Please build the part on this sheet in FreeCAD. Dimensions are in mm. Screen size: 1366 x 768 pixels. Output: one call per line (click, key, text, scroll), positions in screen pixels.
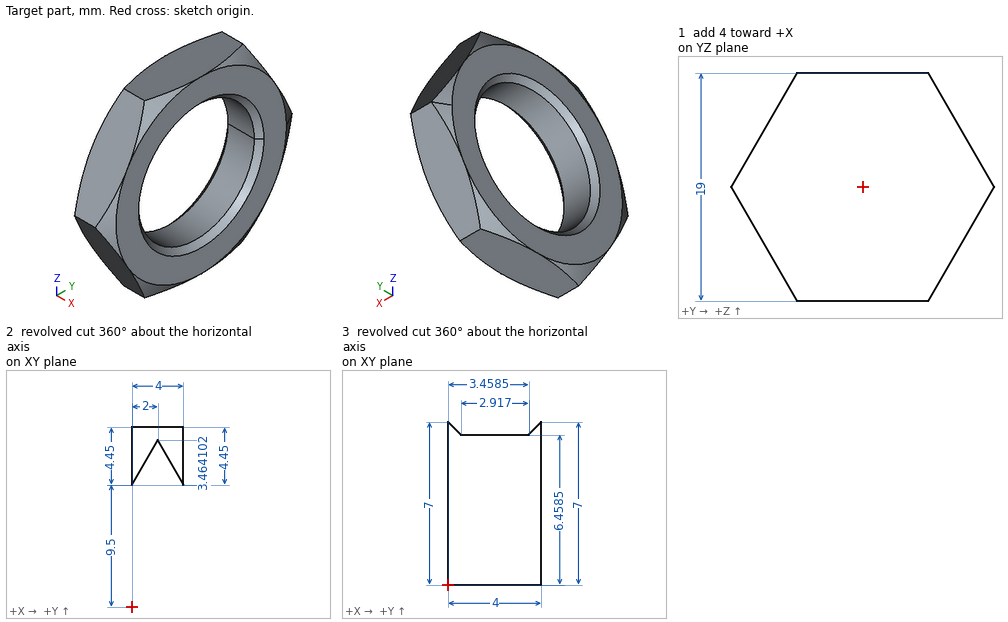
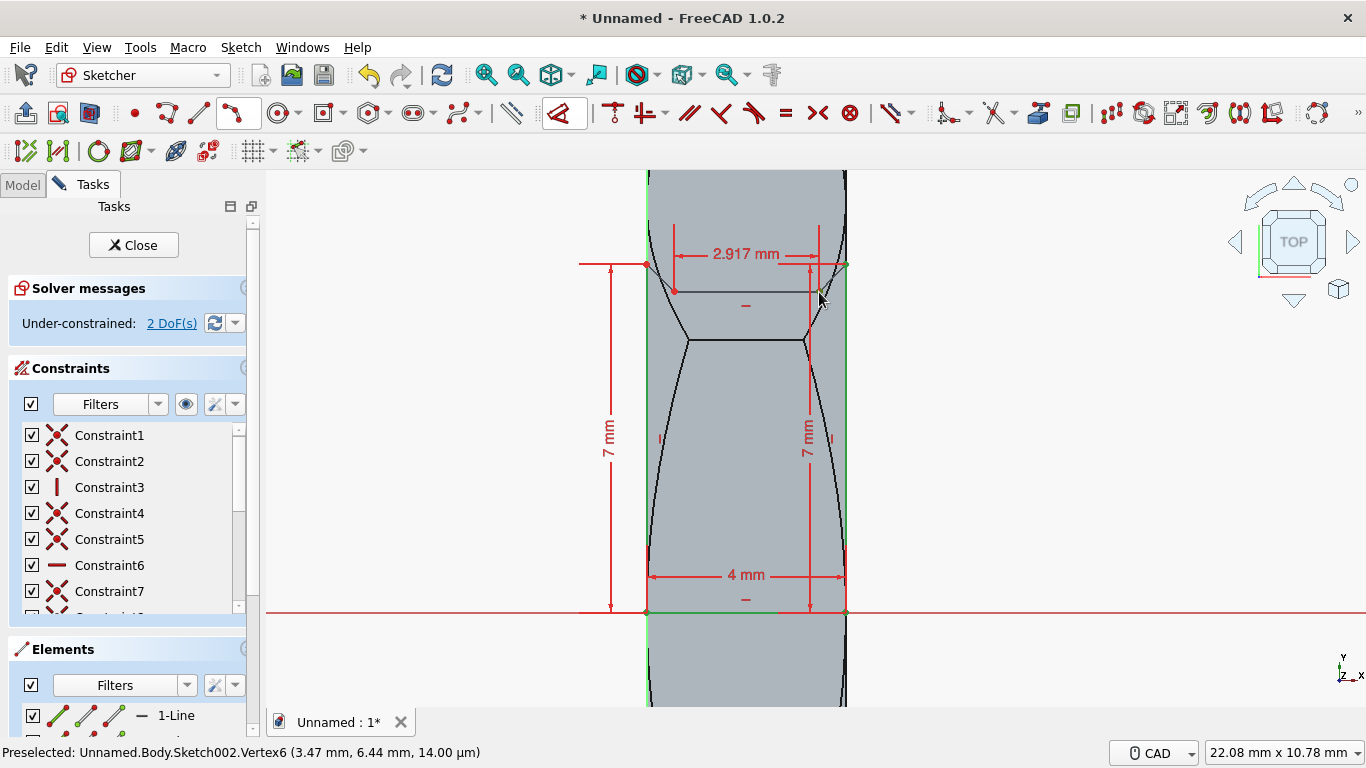
key(l)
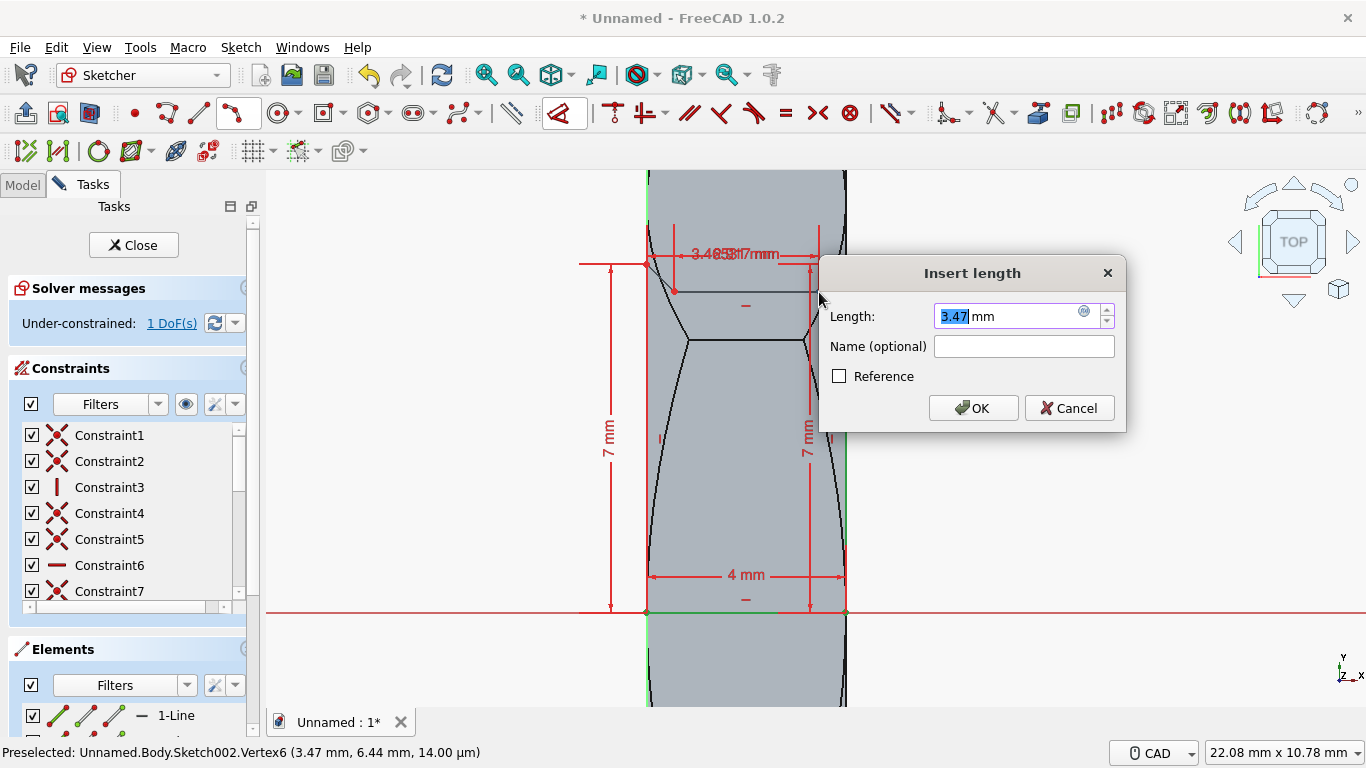
text(3.4585)
key(Return)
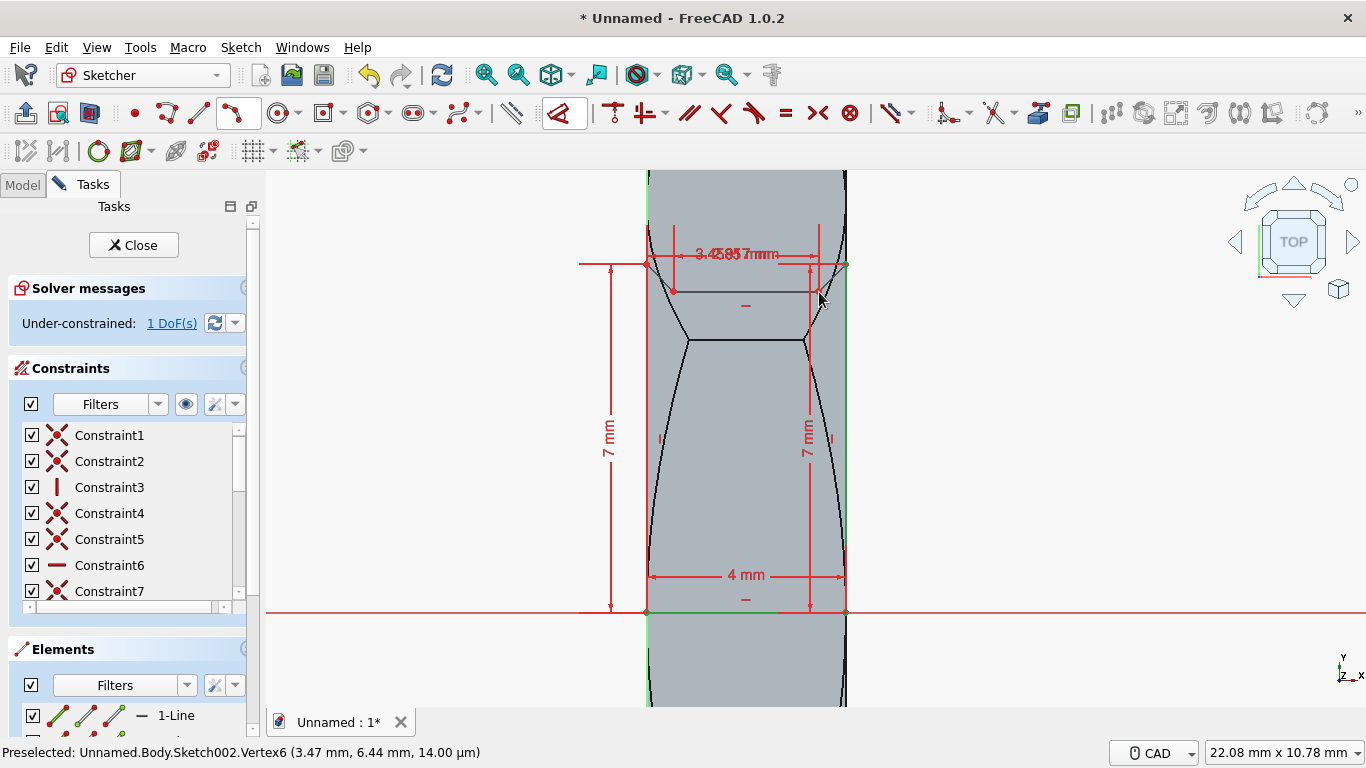
click(819, 292)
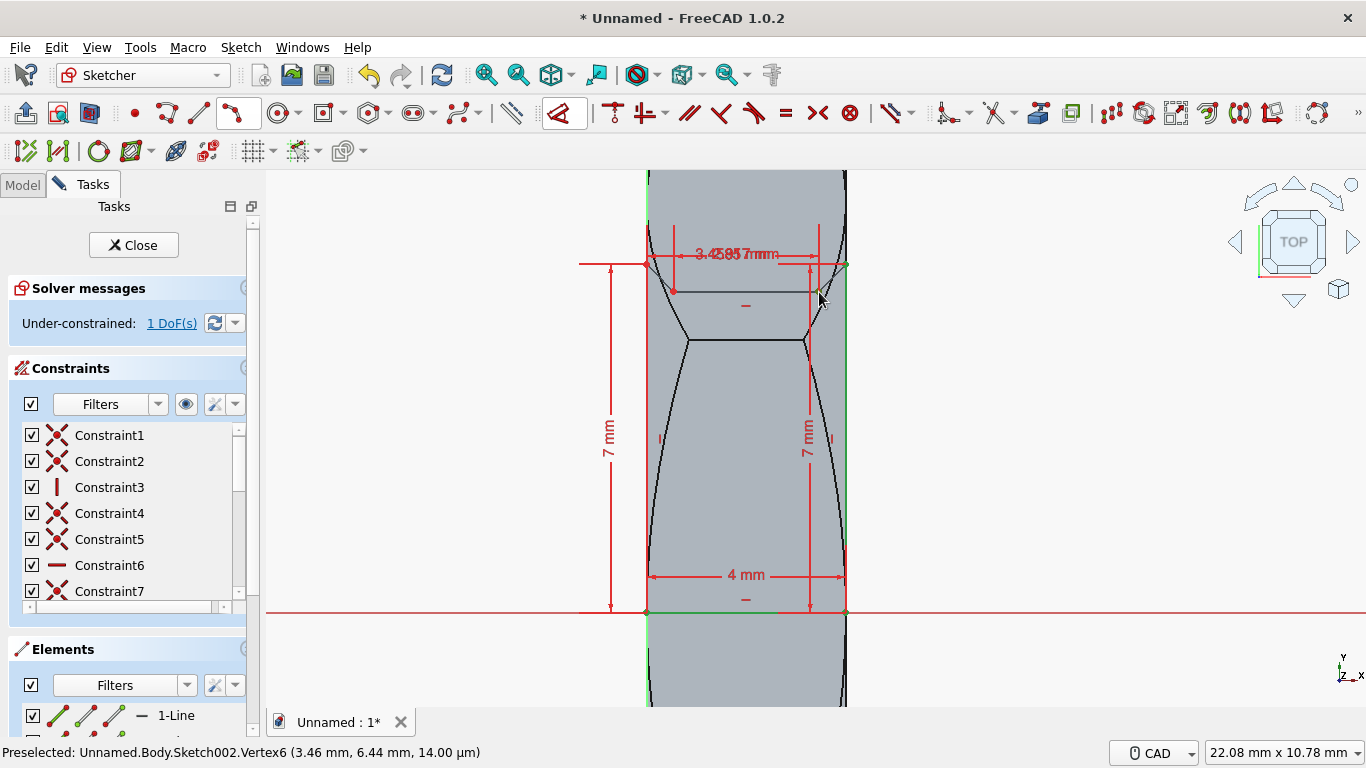
key(i)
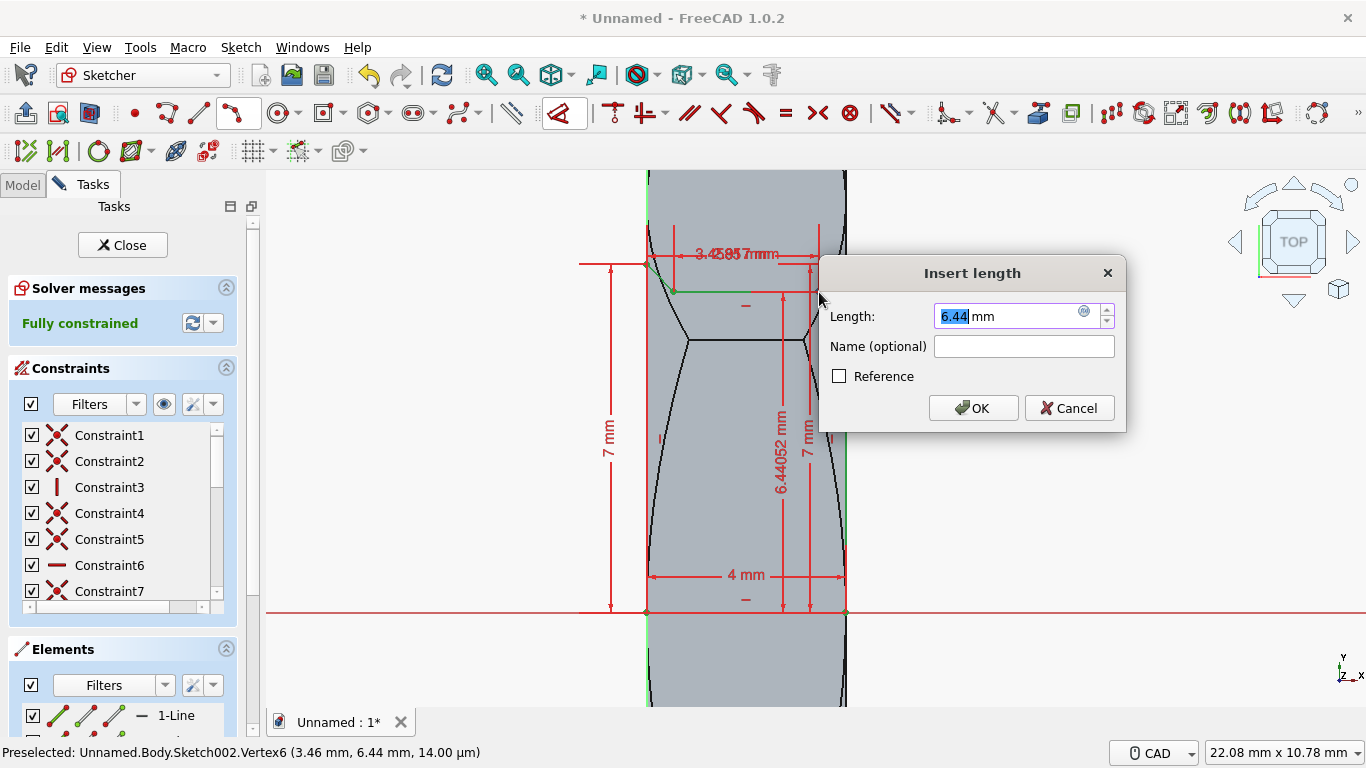
text(6.4585)
key(Return)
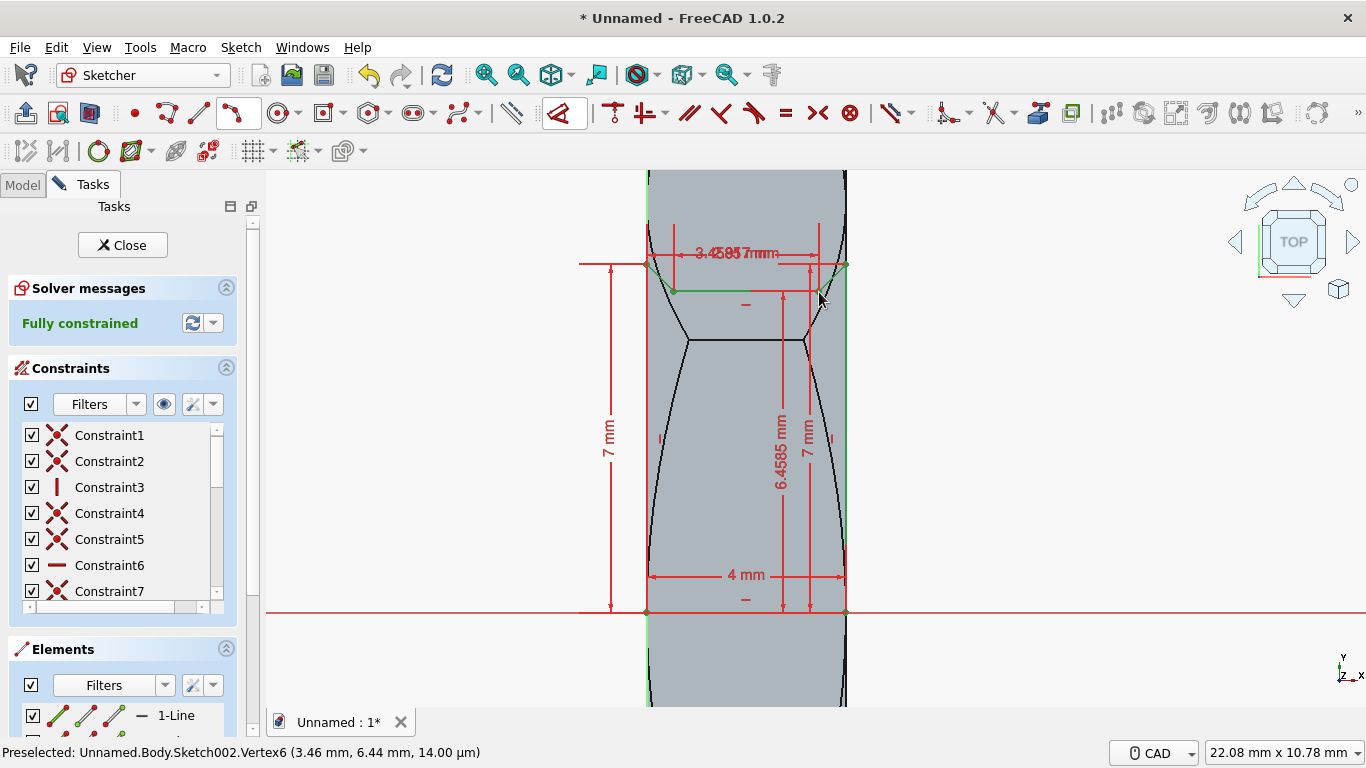
click(123, 245)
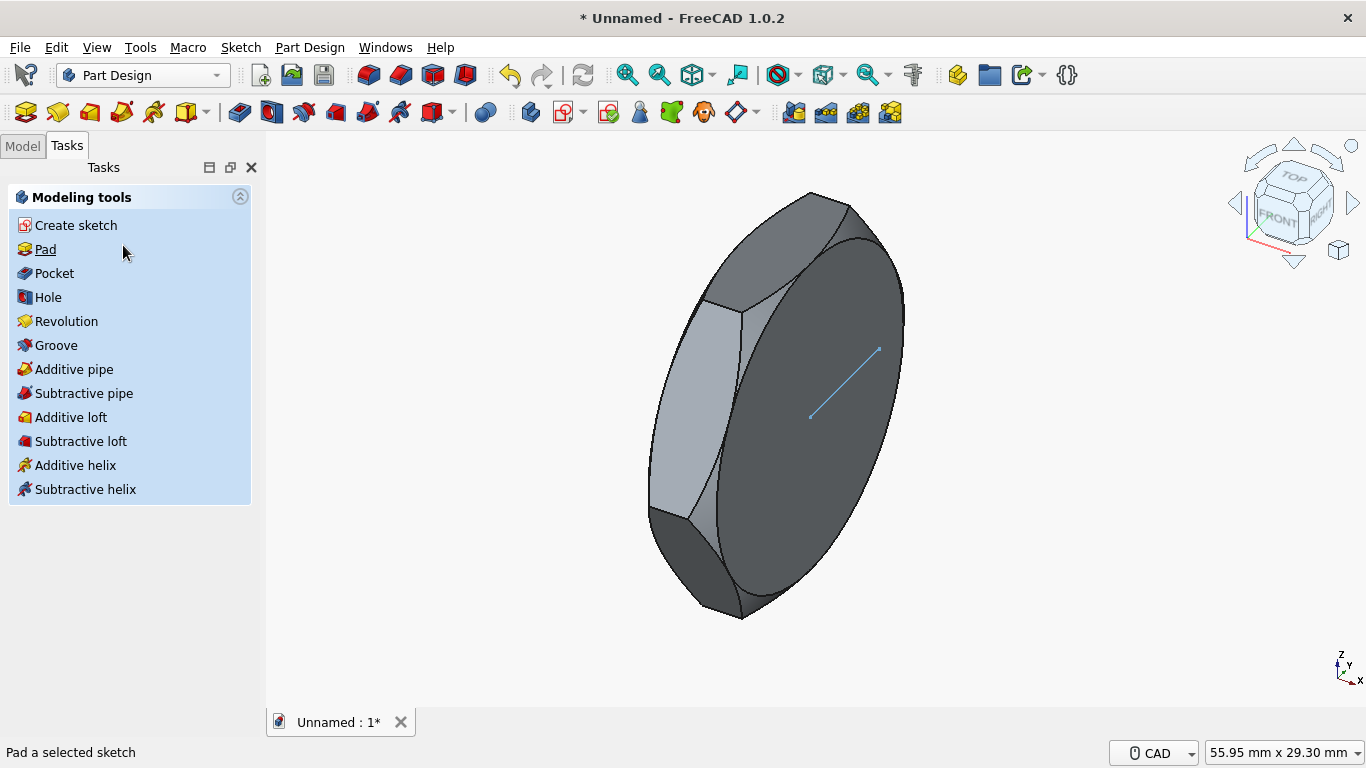
click(304, 112)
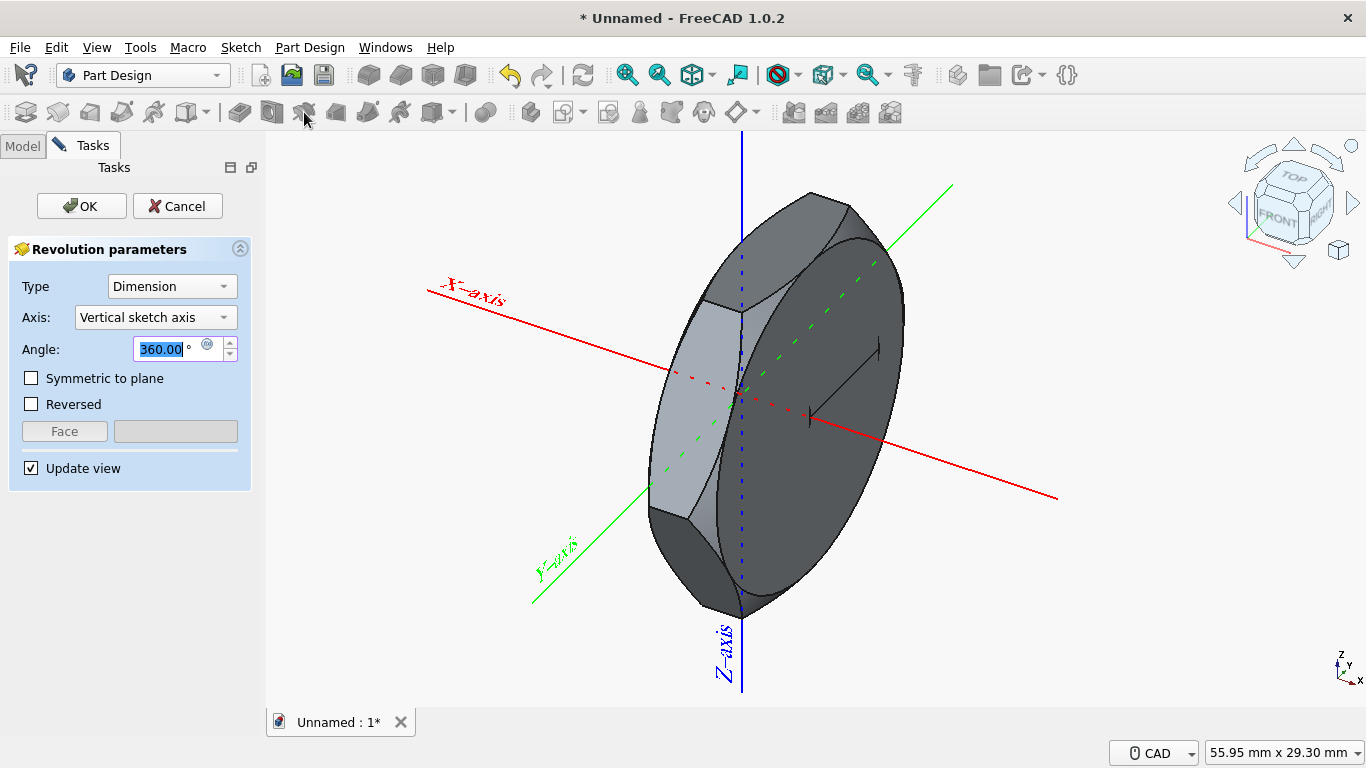
click(156, 318)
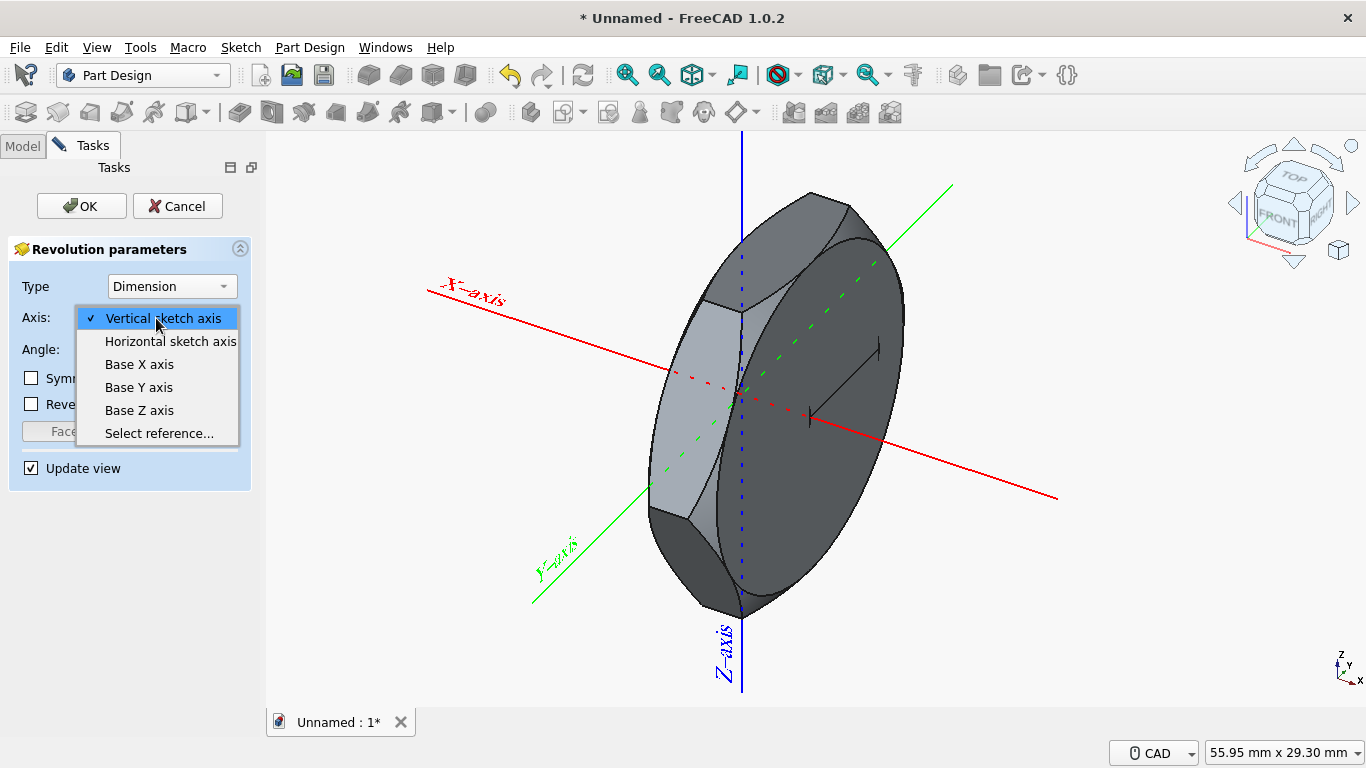
click(156, 342)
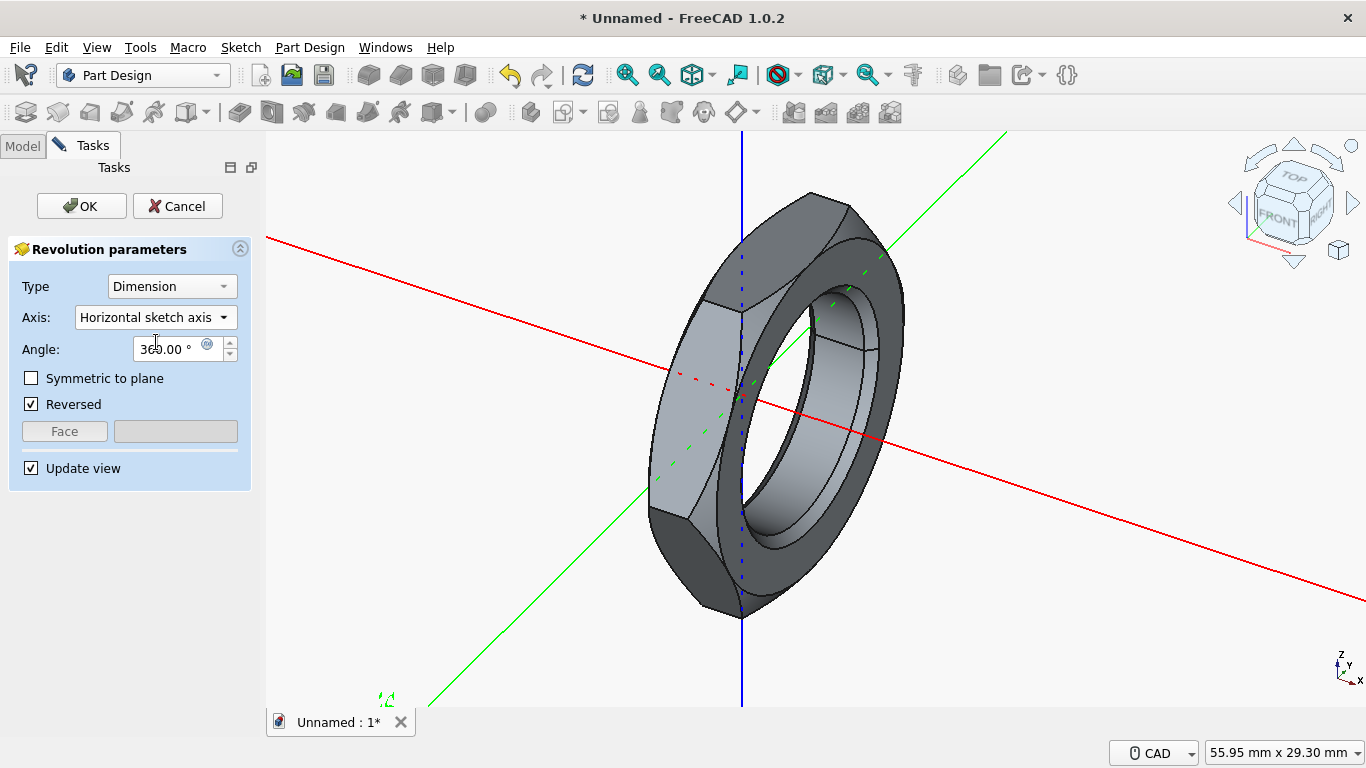
click(82, 206)